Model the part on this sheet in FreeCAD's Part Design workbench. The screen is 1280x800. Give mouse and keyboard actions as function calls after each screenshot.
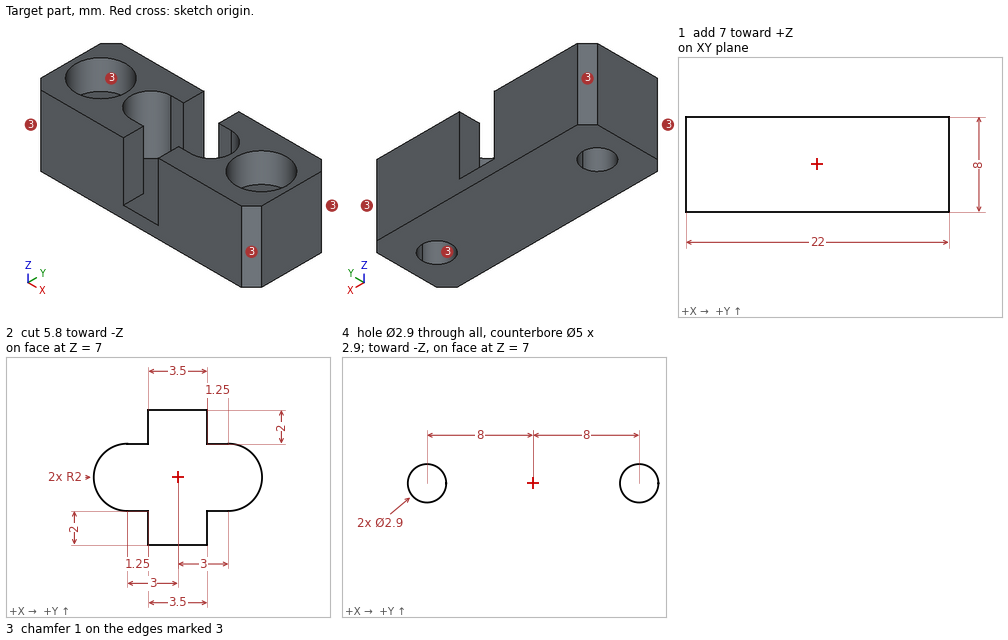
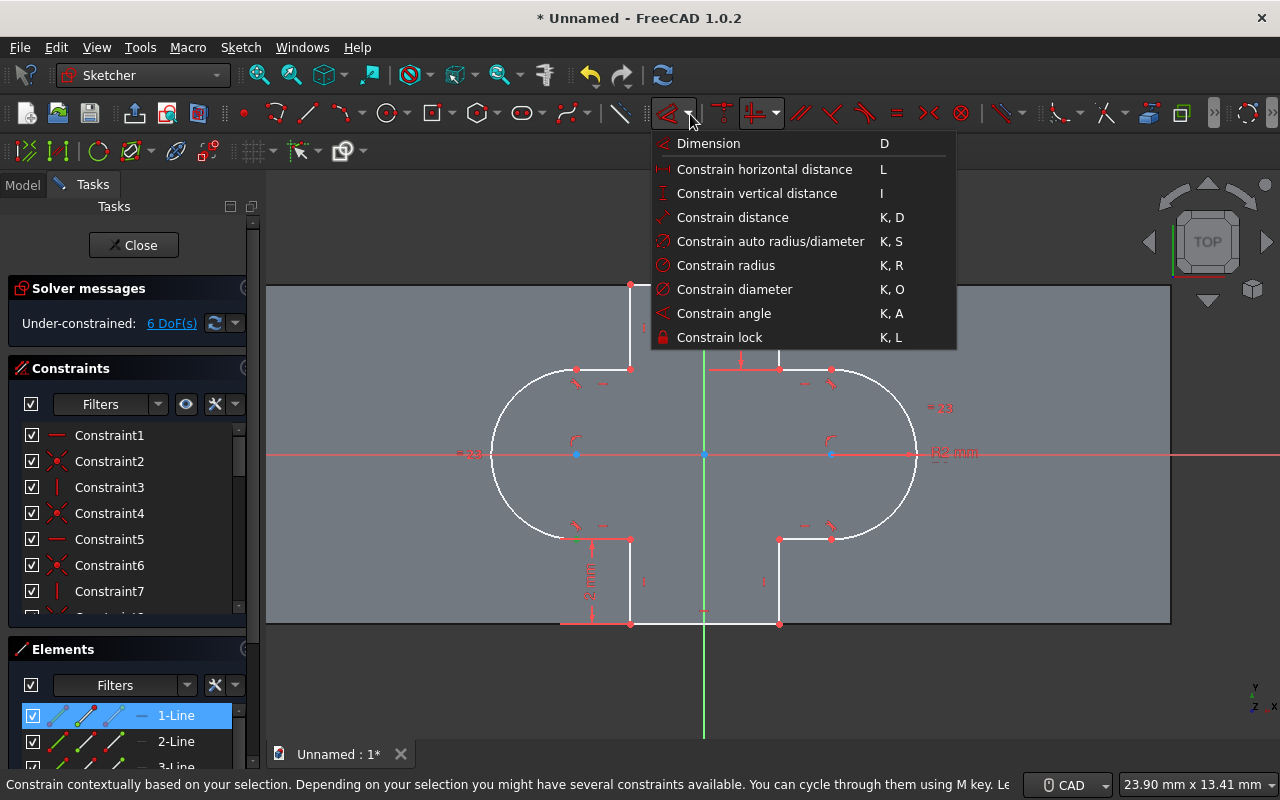
click(804, 169)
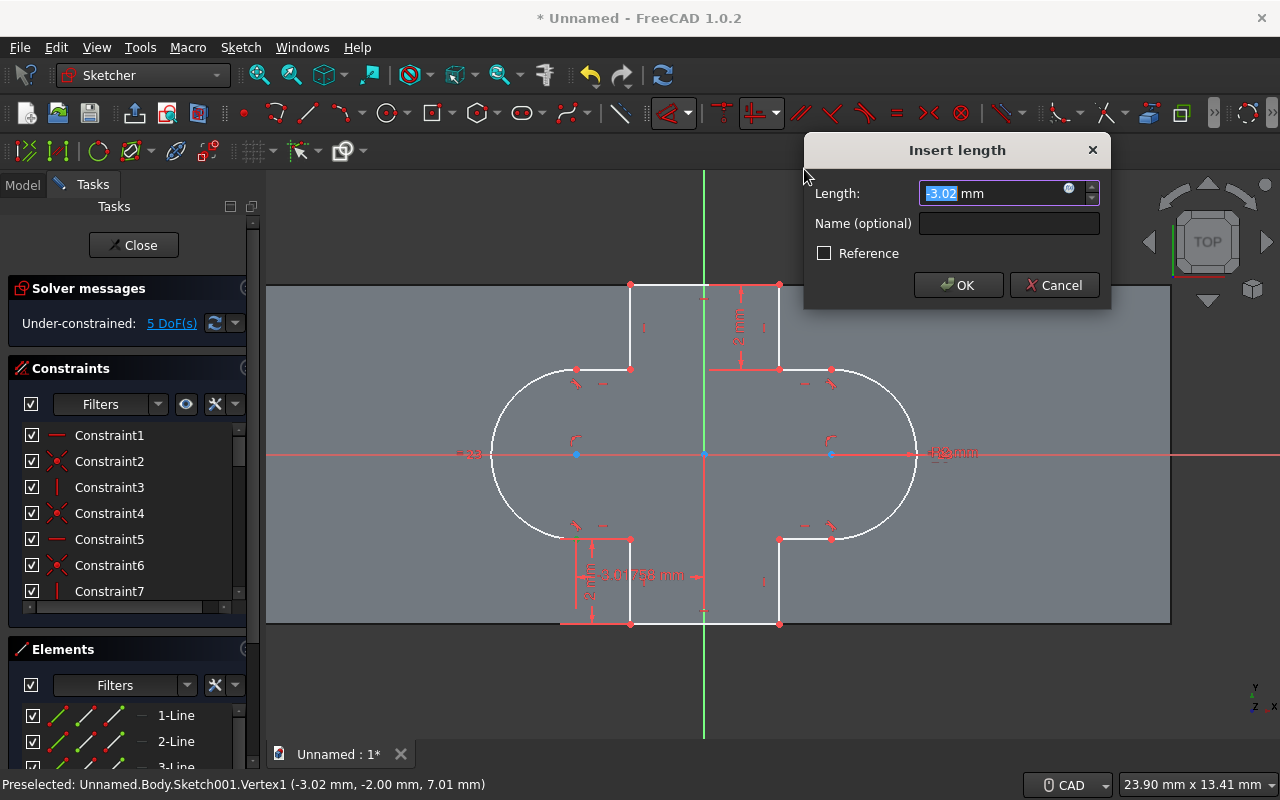
text(-3)
key(Return)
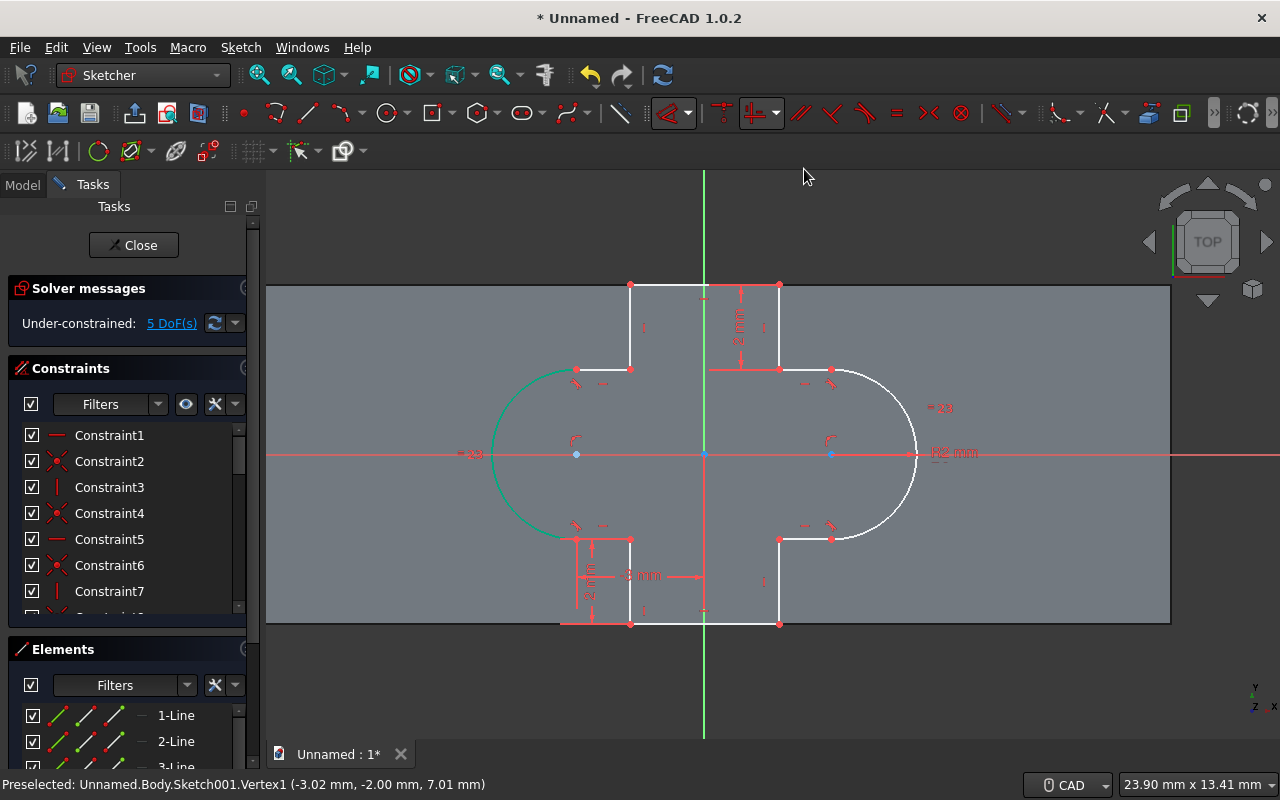
click(832, 539)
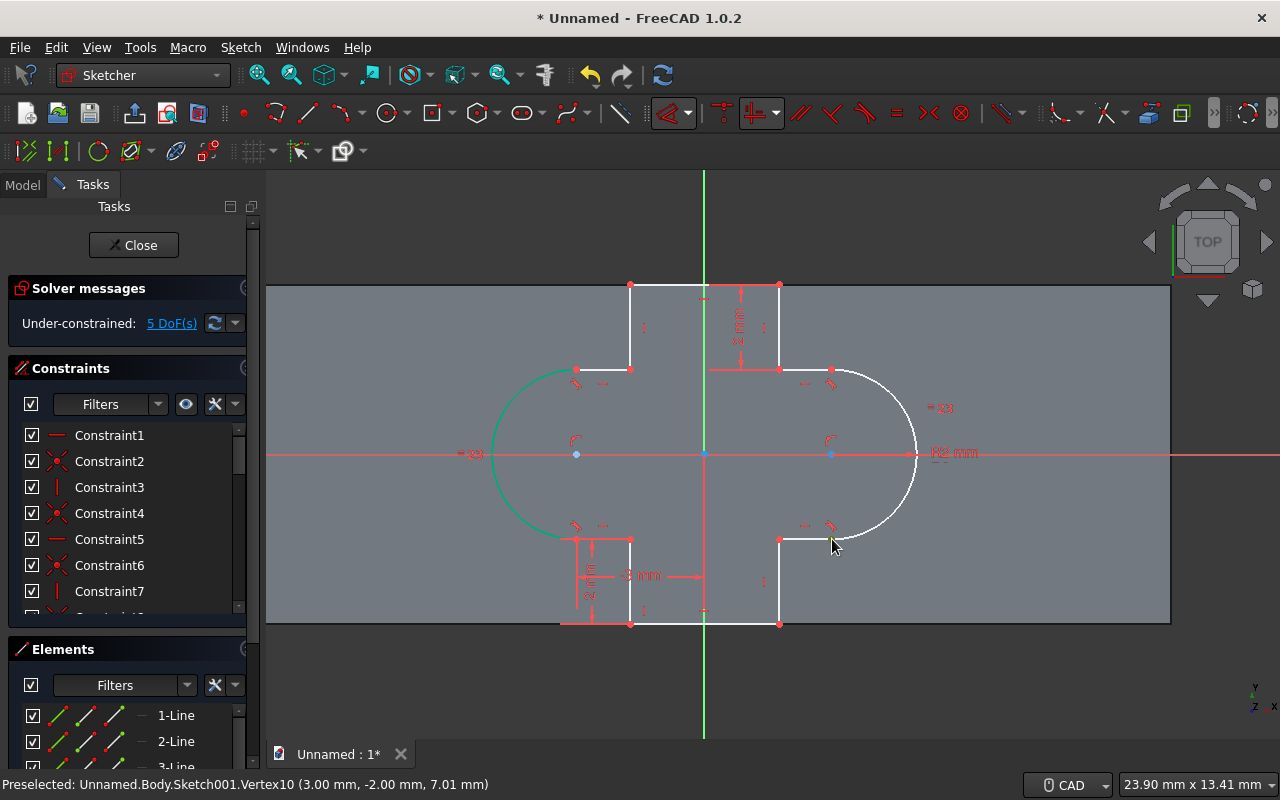
click(690, 114)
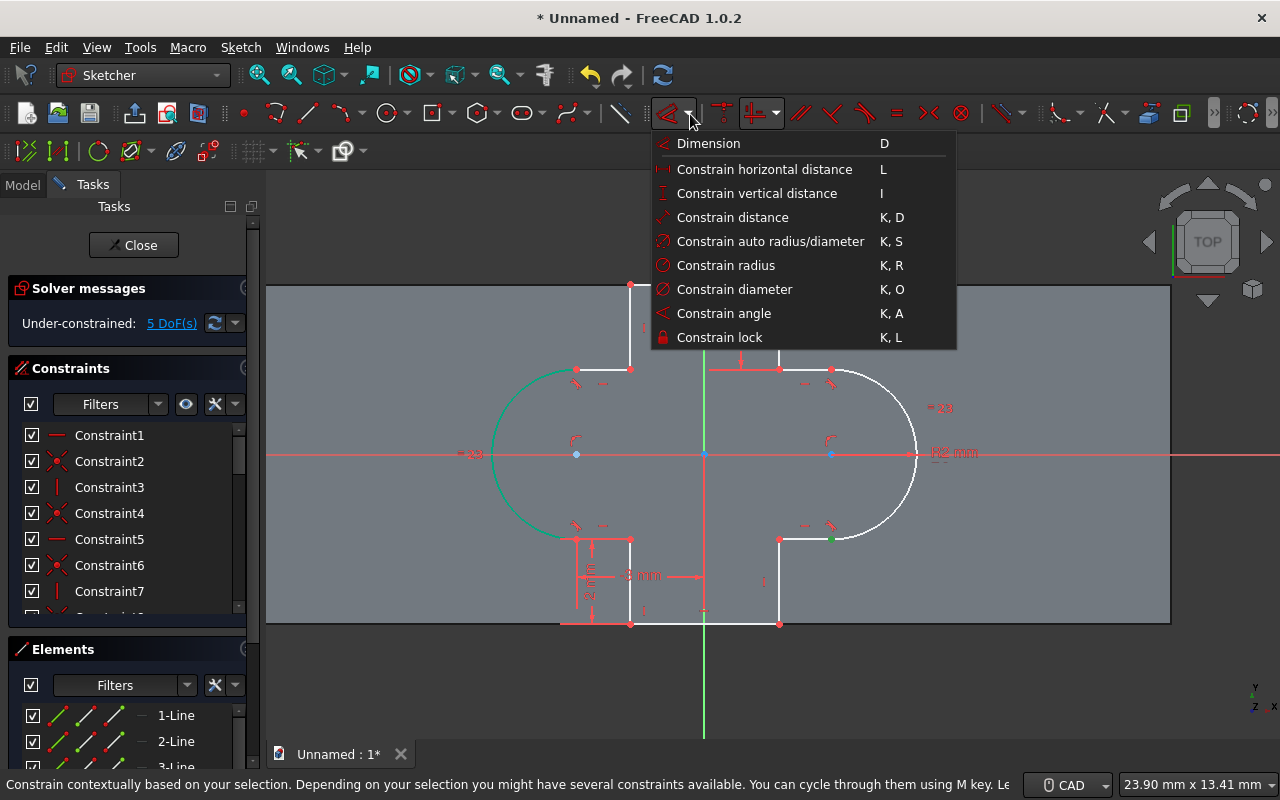
click(804, 169)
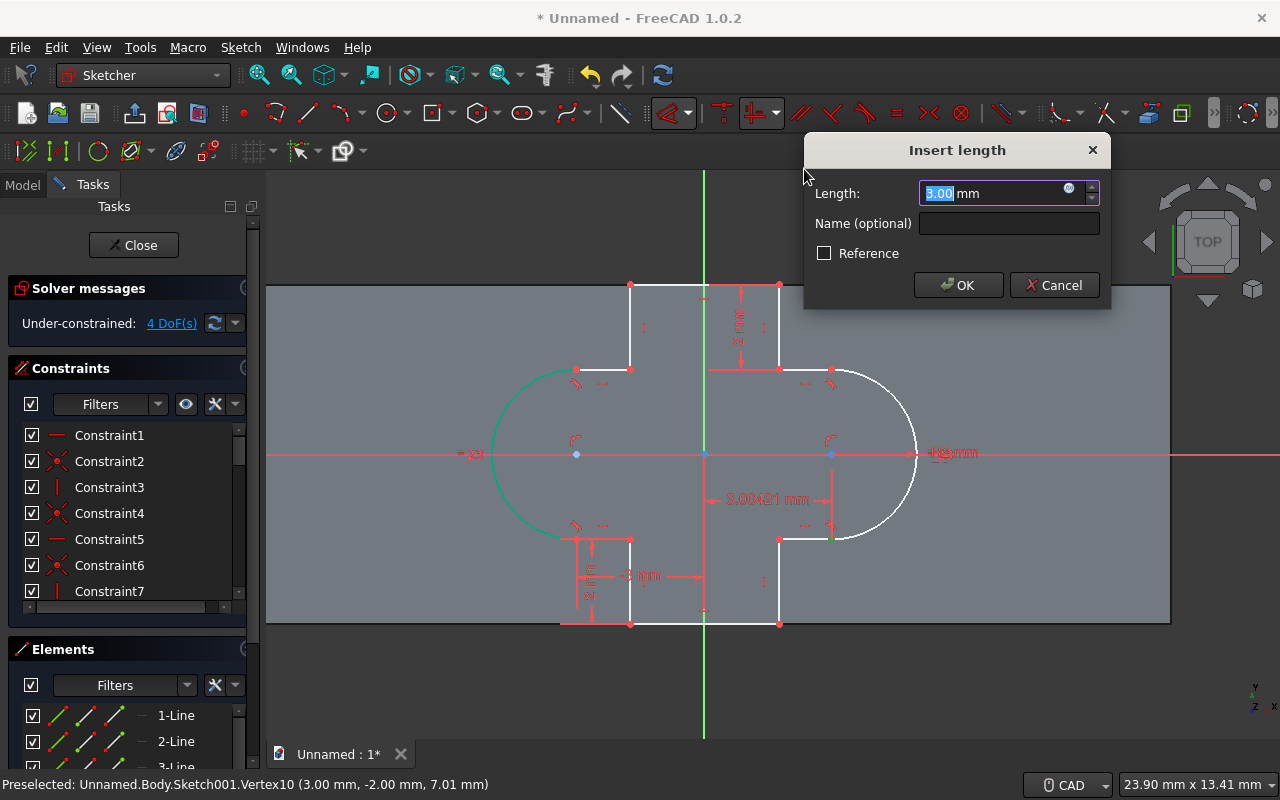
text(3)
key(Return)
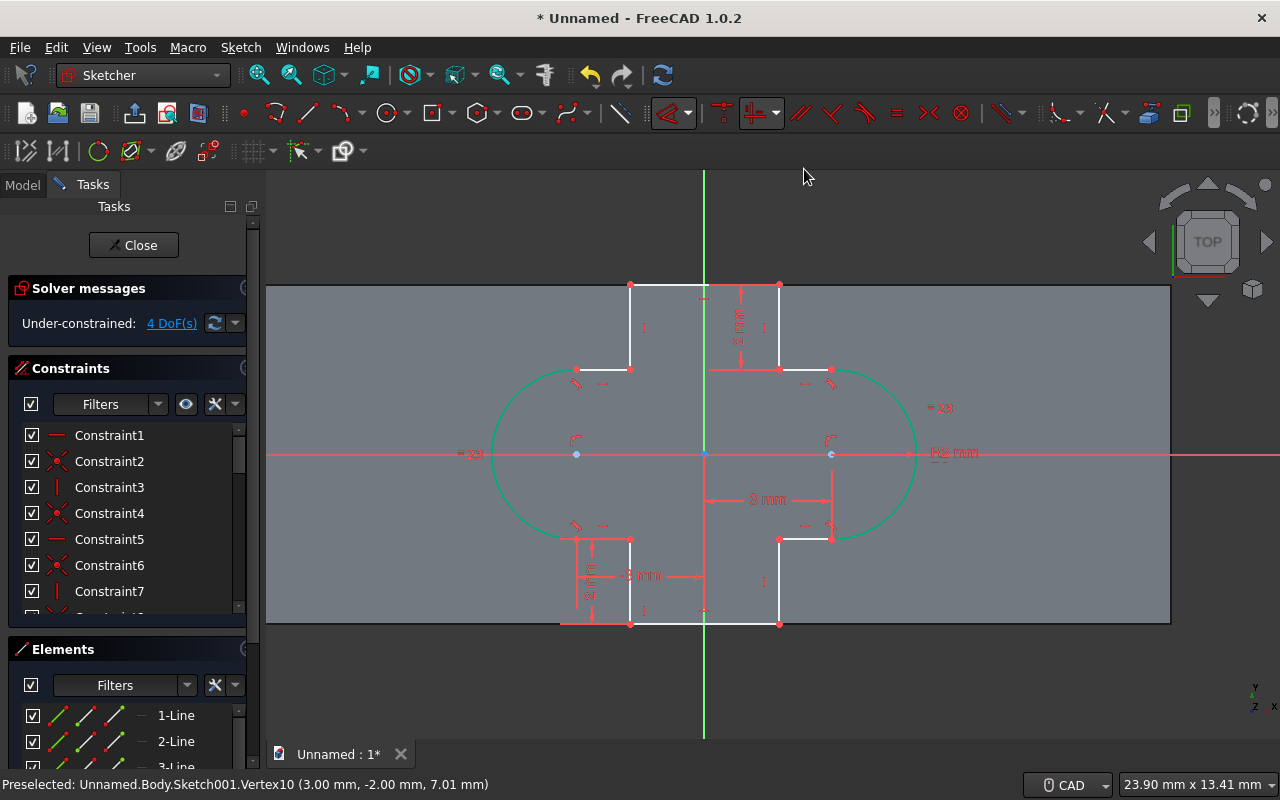
click(675, 624)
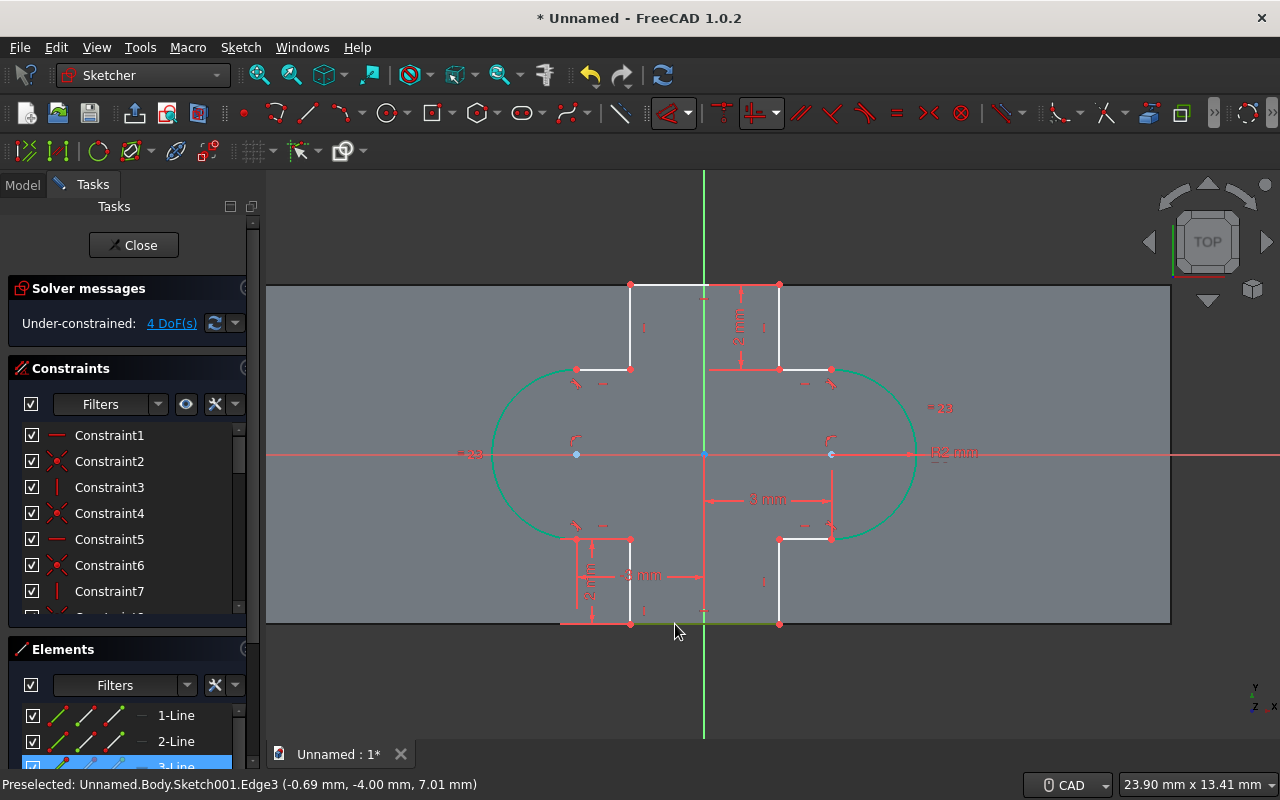
click(690, 114)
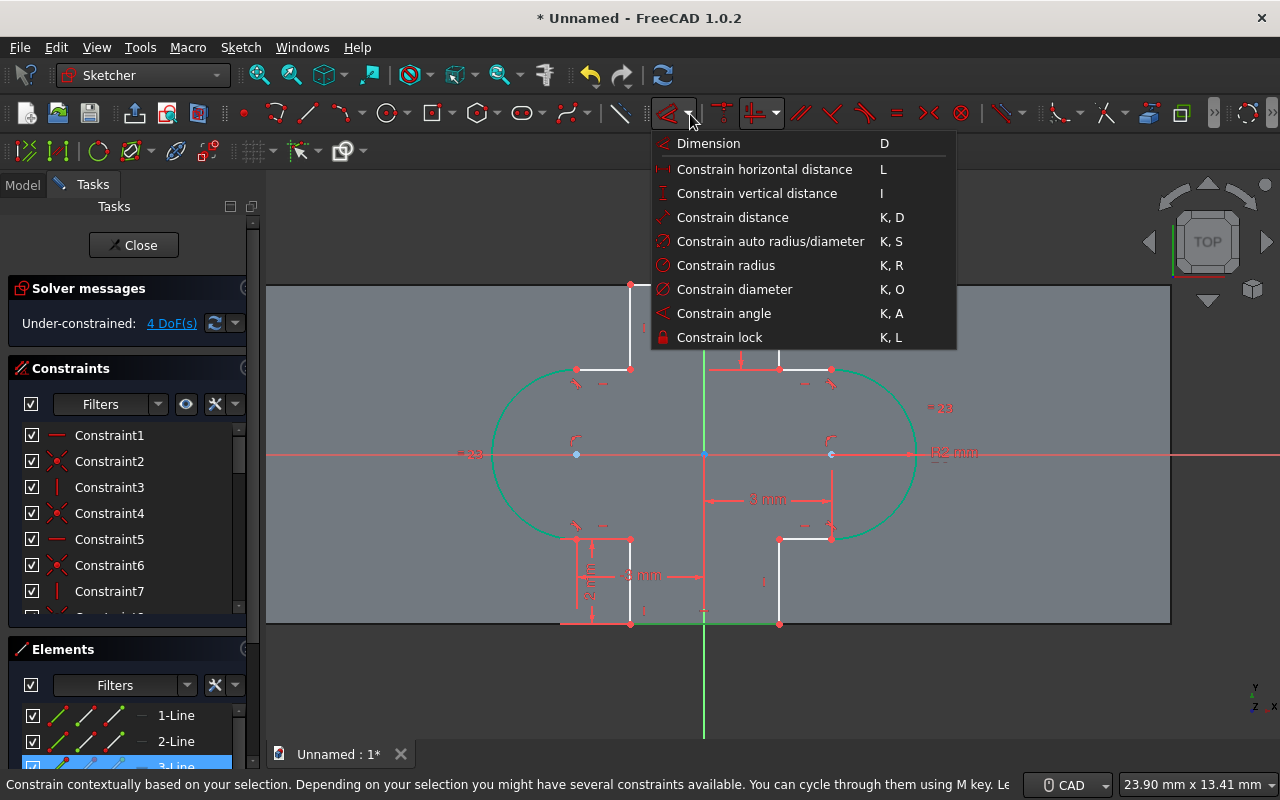
click(804, 169)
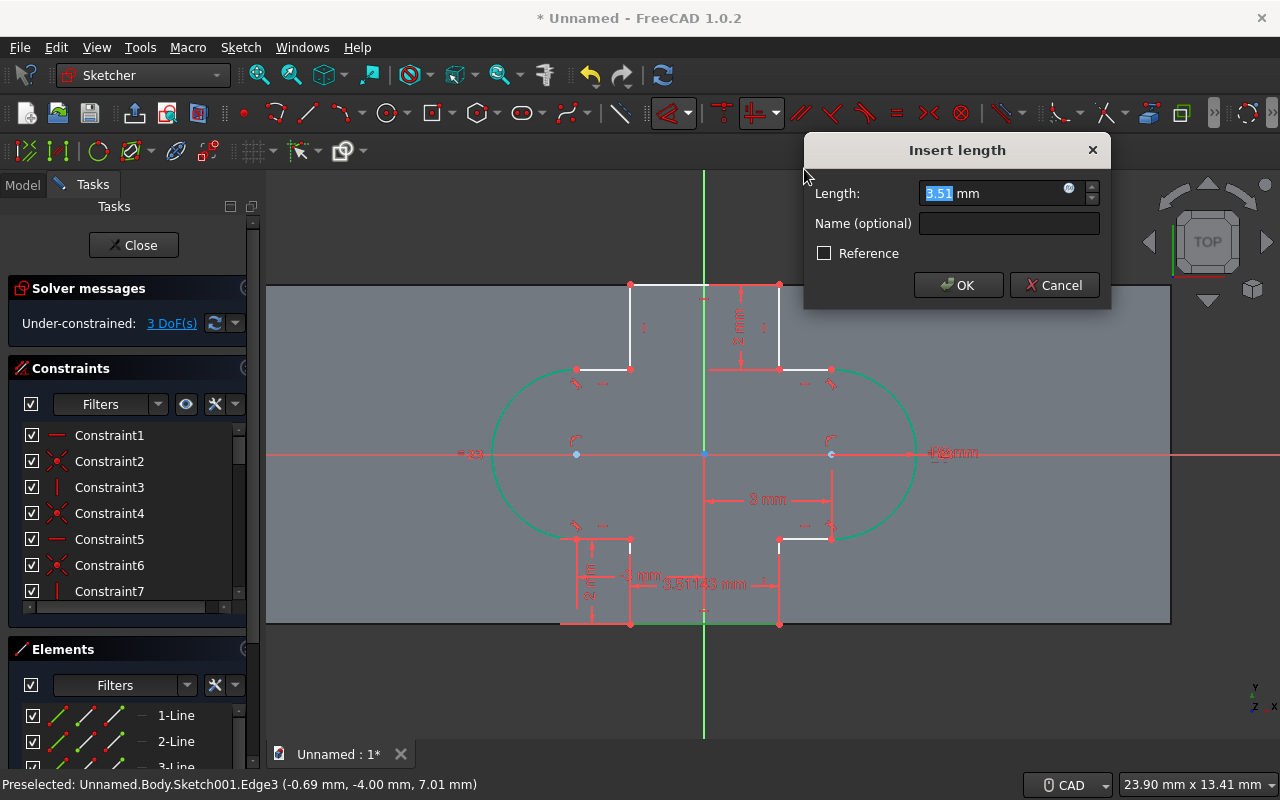
text(3.5)
key(Return)